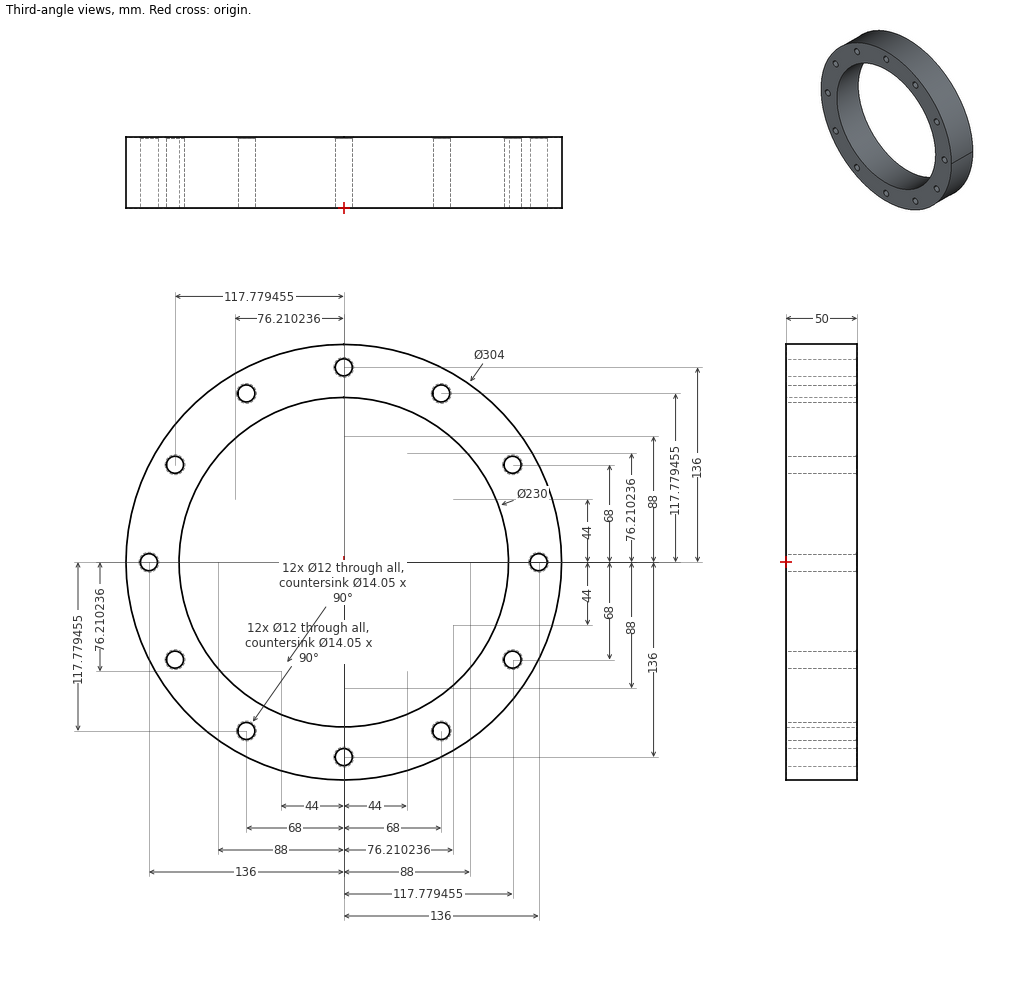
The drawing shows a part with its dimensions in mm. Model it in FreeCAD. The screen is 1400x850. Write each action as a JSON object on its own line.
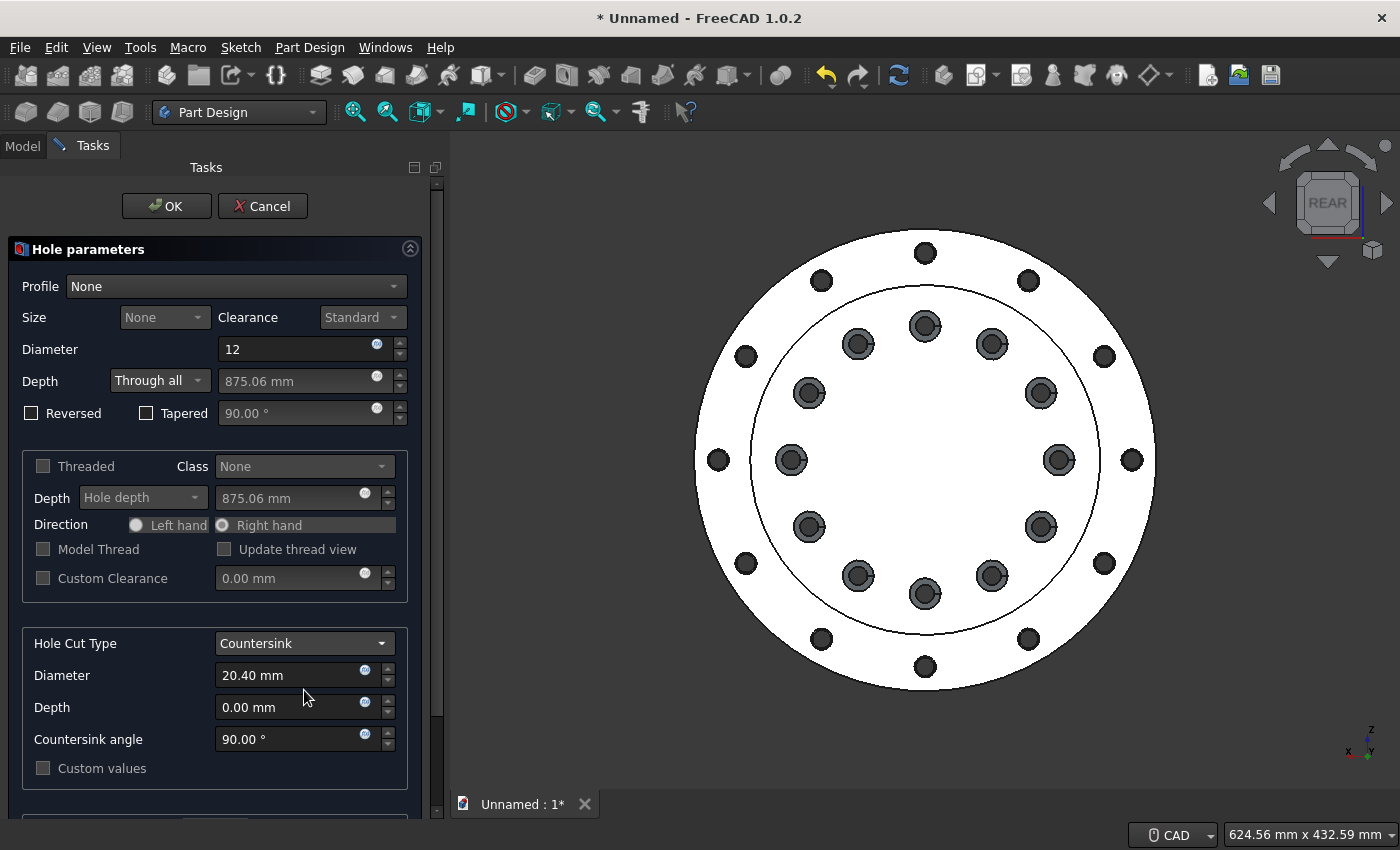
{"action": "triple_click", "coordinate": [298, 675]}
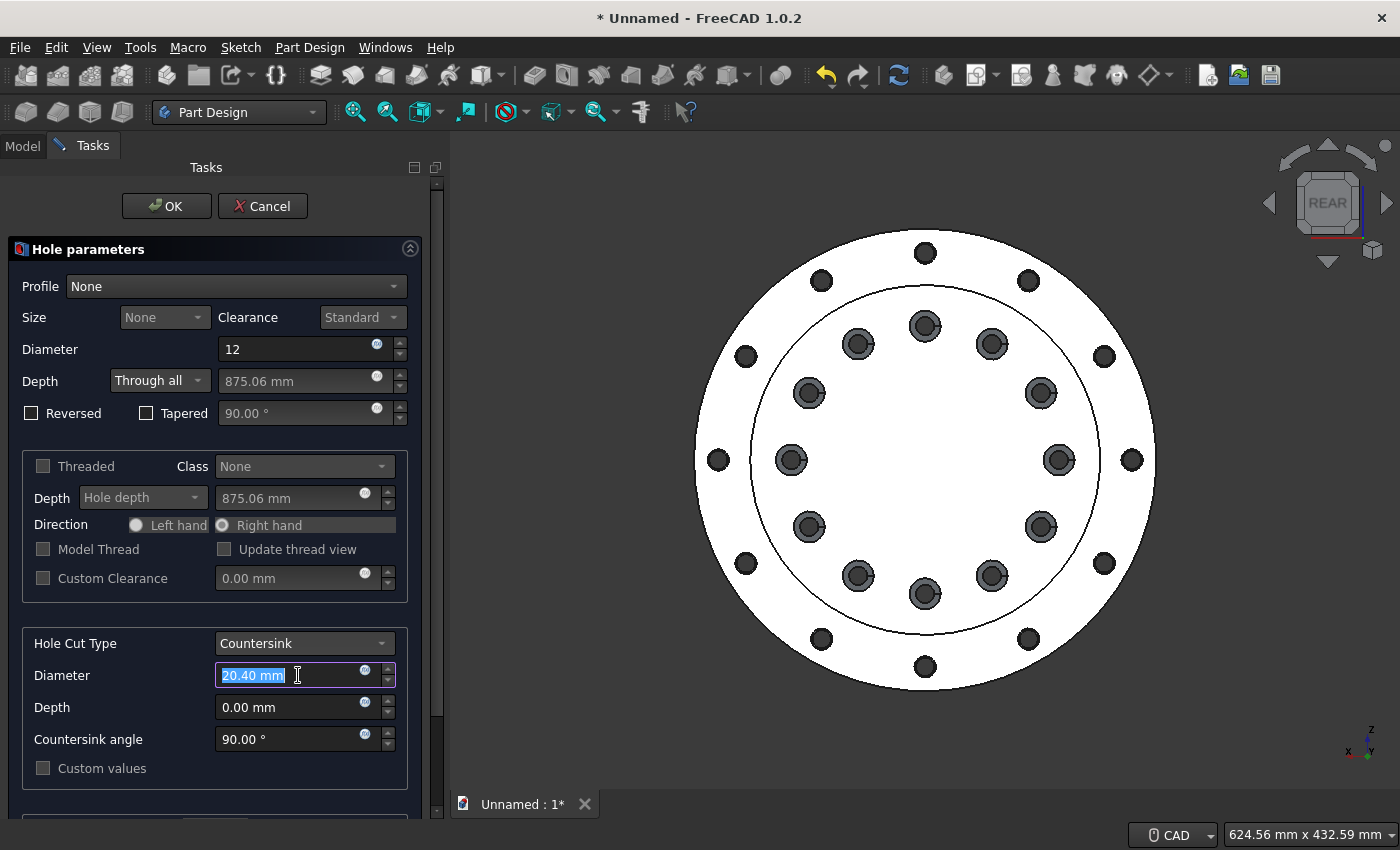
{"action": "type", "text": "14.05"}
{"action": "key", "text": "Tab"}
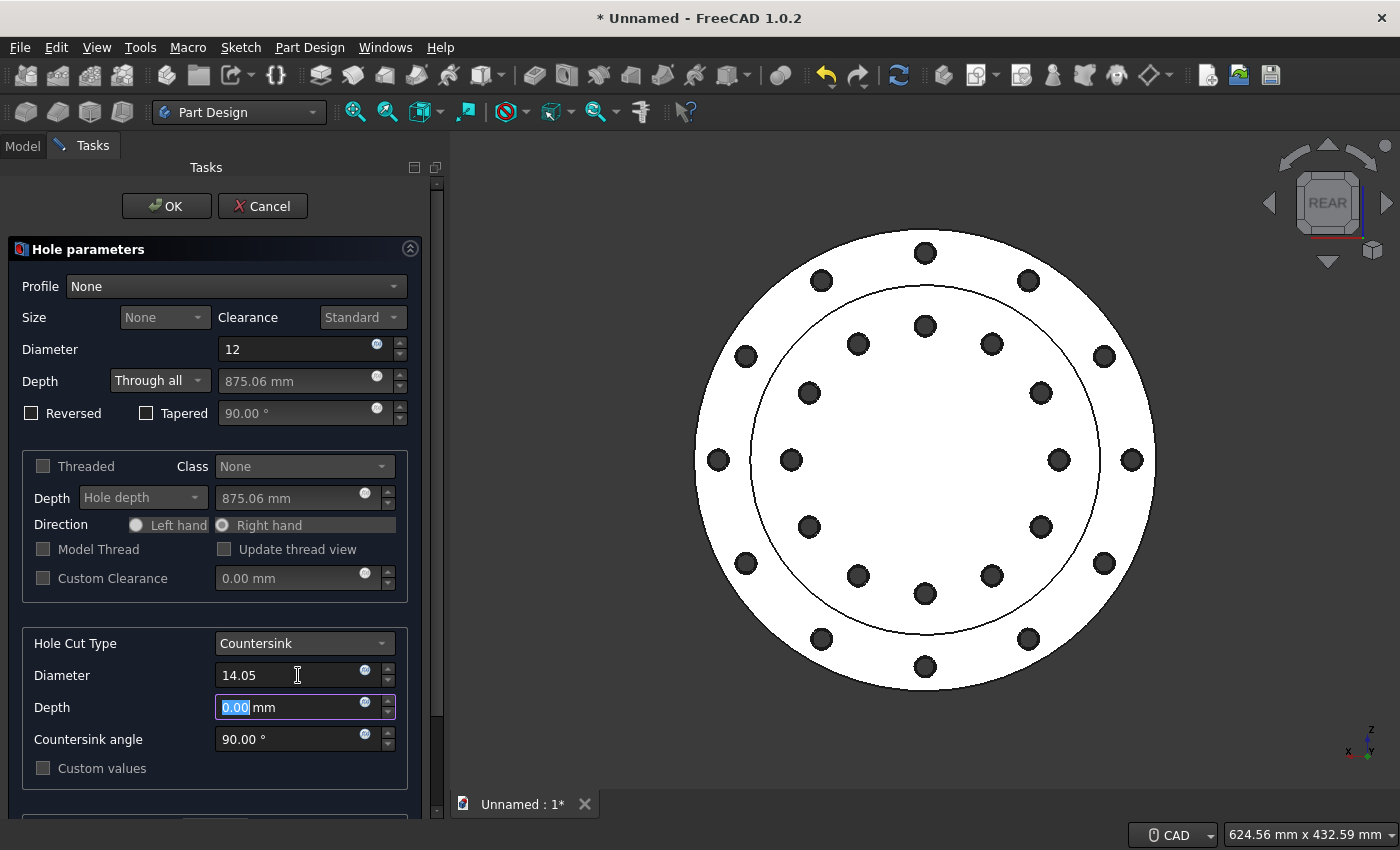
{"action": "left_click", "coordinate": [167, 206]}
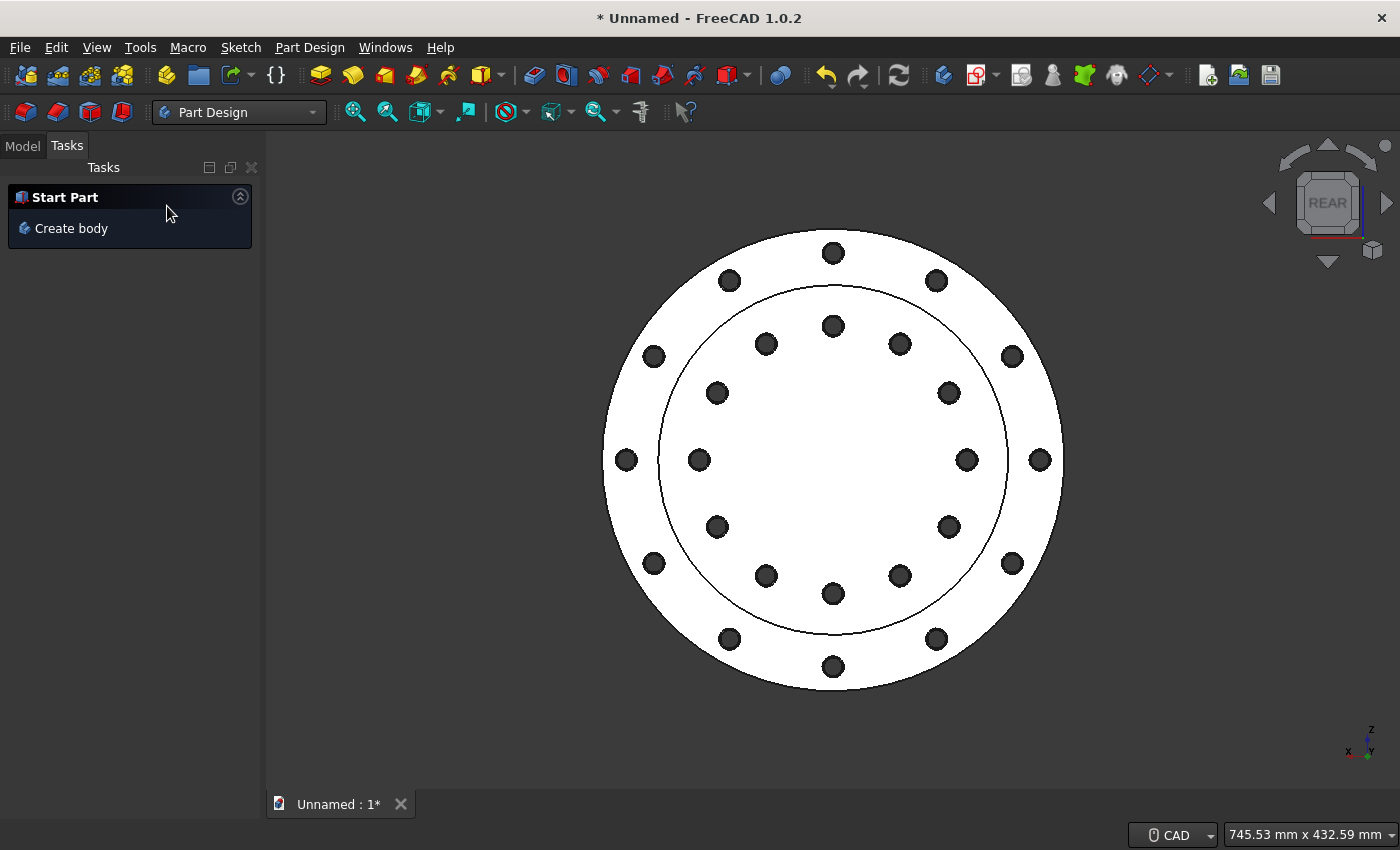
{"action": "left_click", "coordinate": [833, 459]}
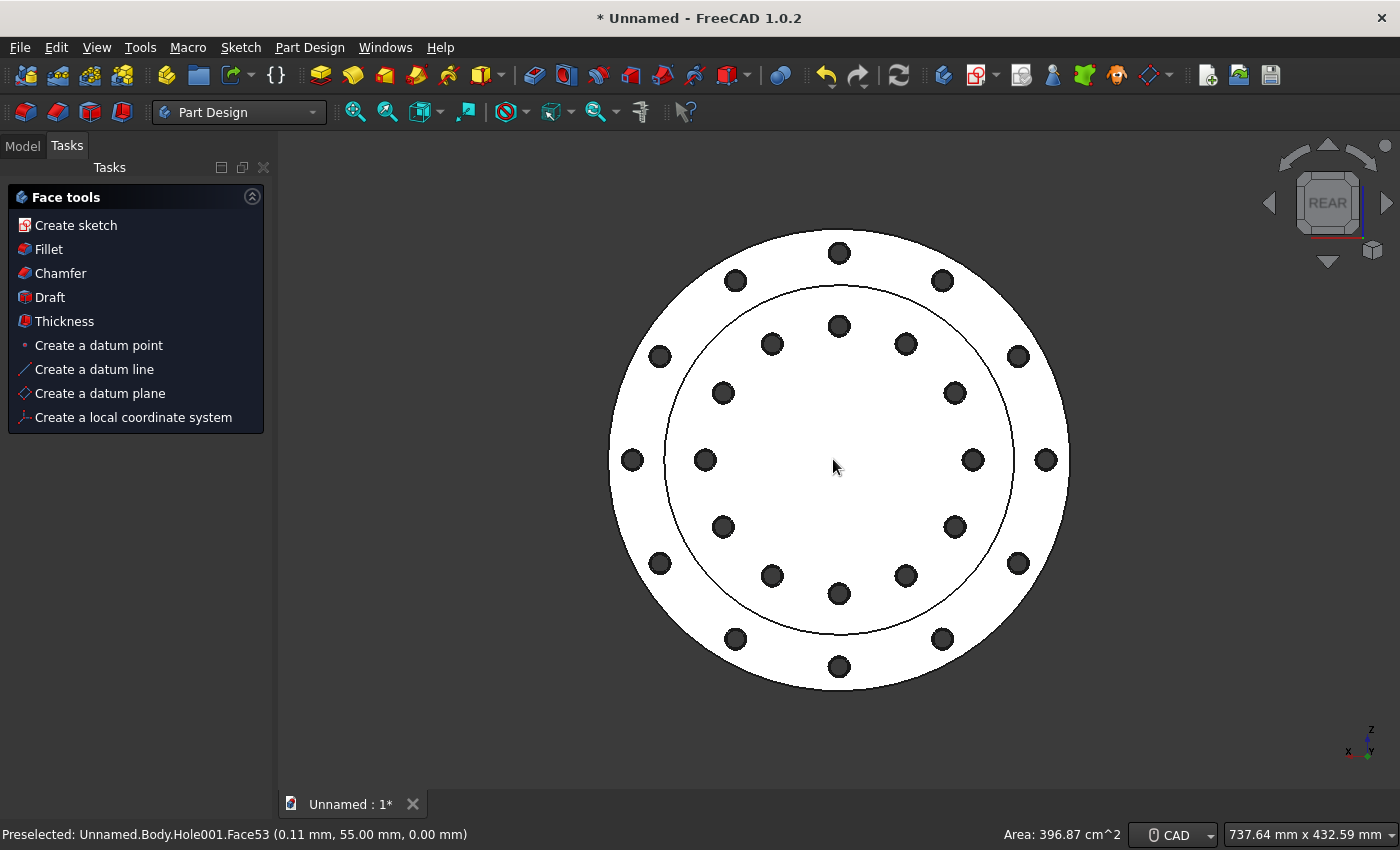
{"action": "left_click", "coordinate": [976, 76]}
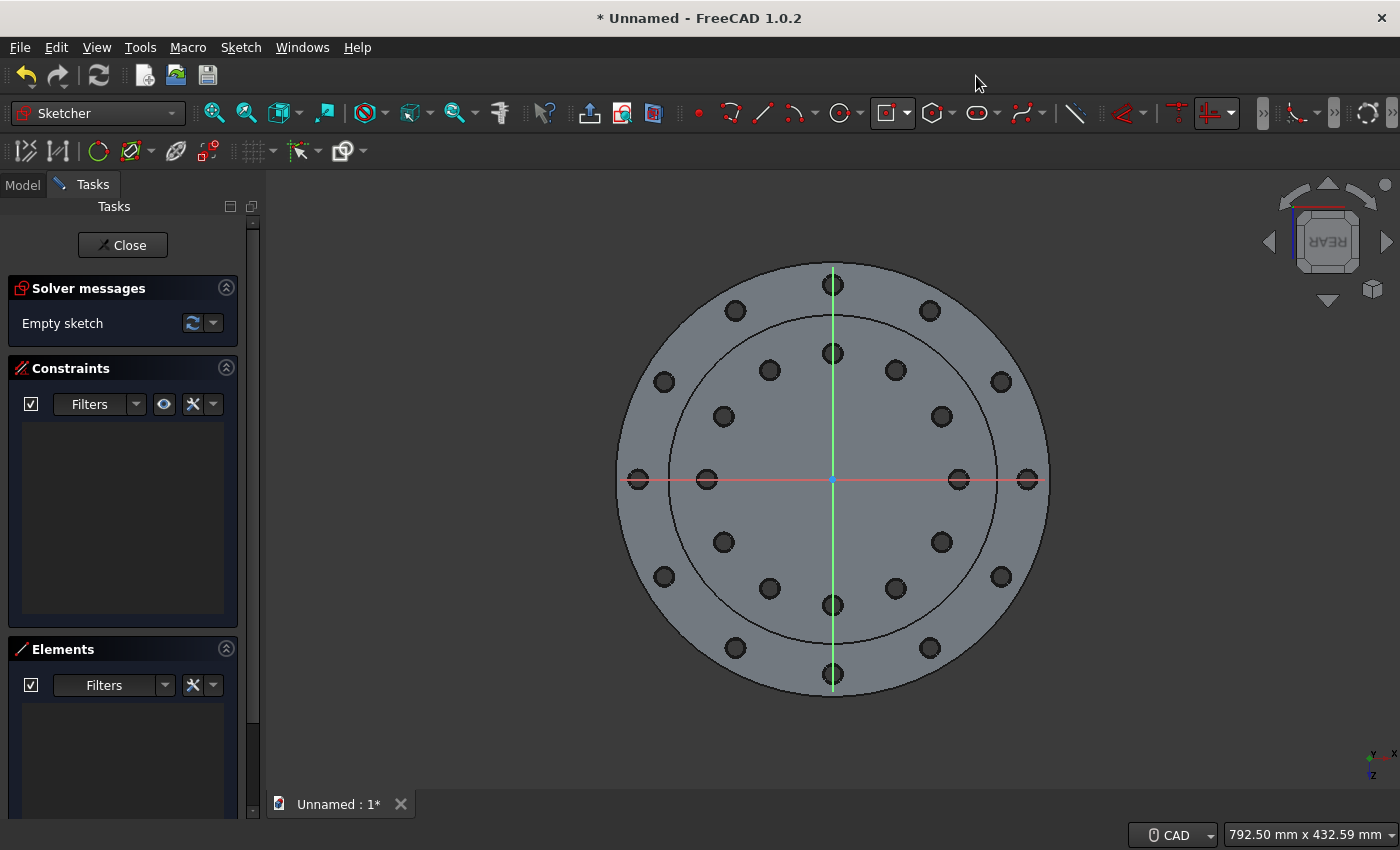
{"action": "key", "text": "g c"}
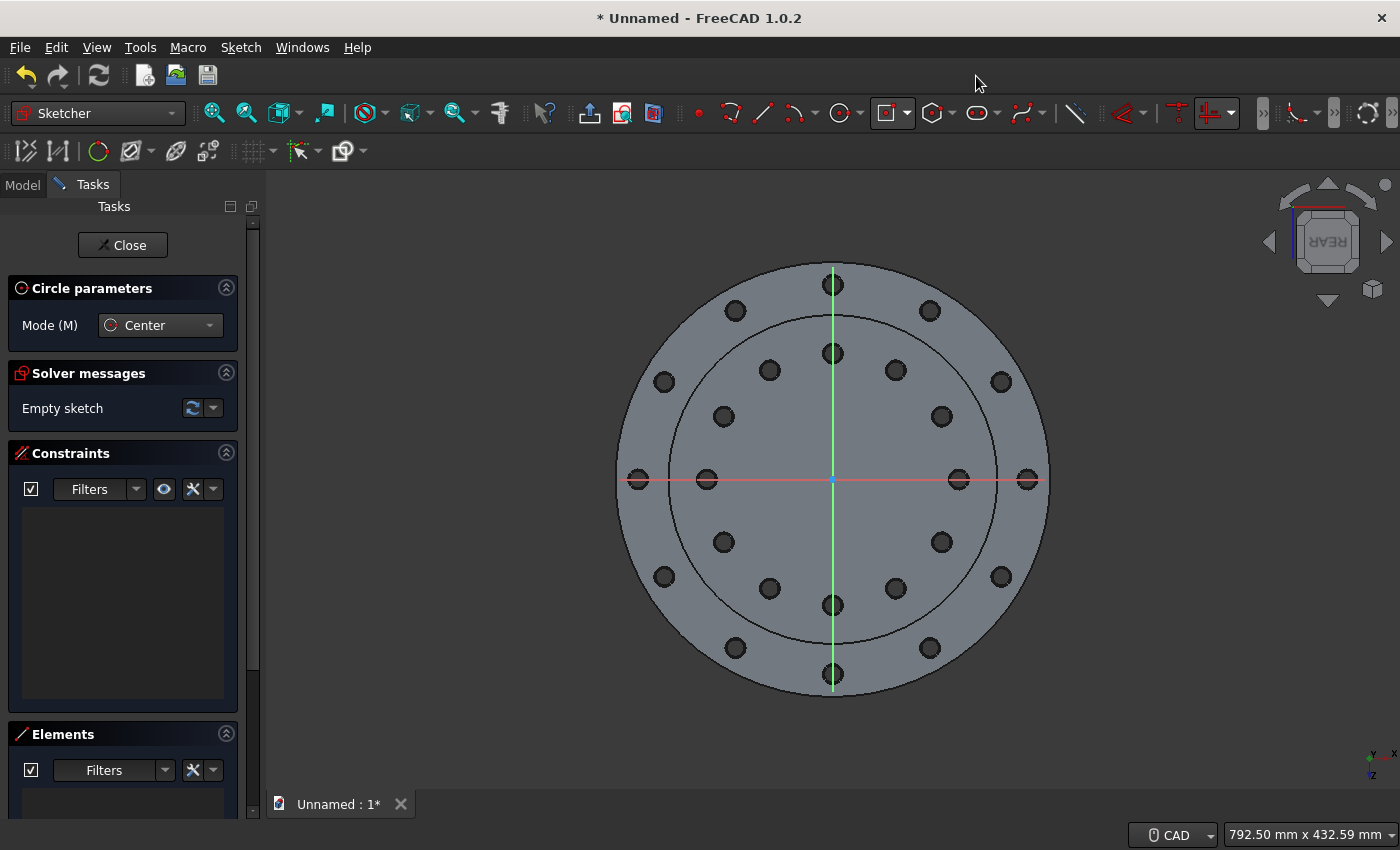
{"action": "left_click", "coordinate": [833, 479]}
{"action": "left_click", "coordinate": [949, 363]}
{"action": "key", "text": "Escape"}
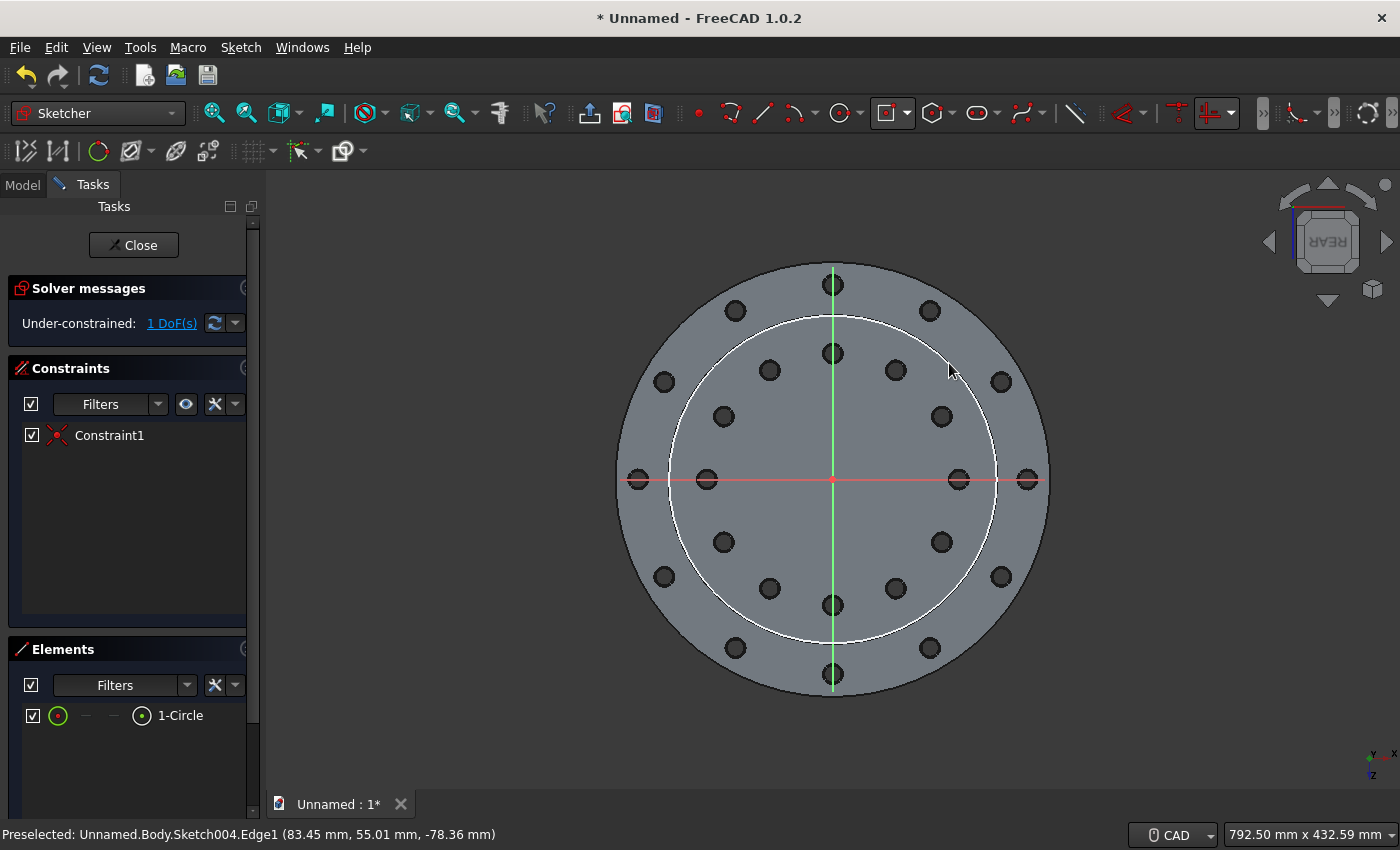
{"action": "left_click", "coordinate": [1122, 114]}